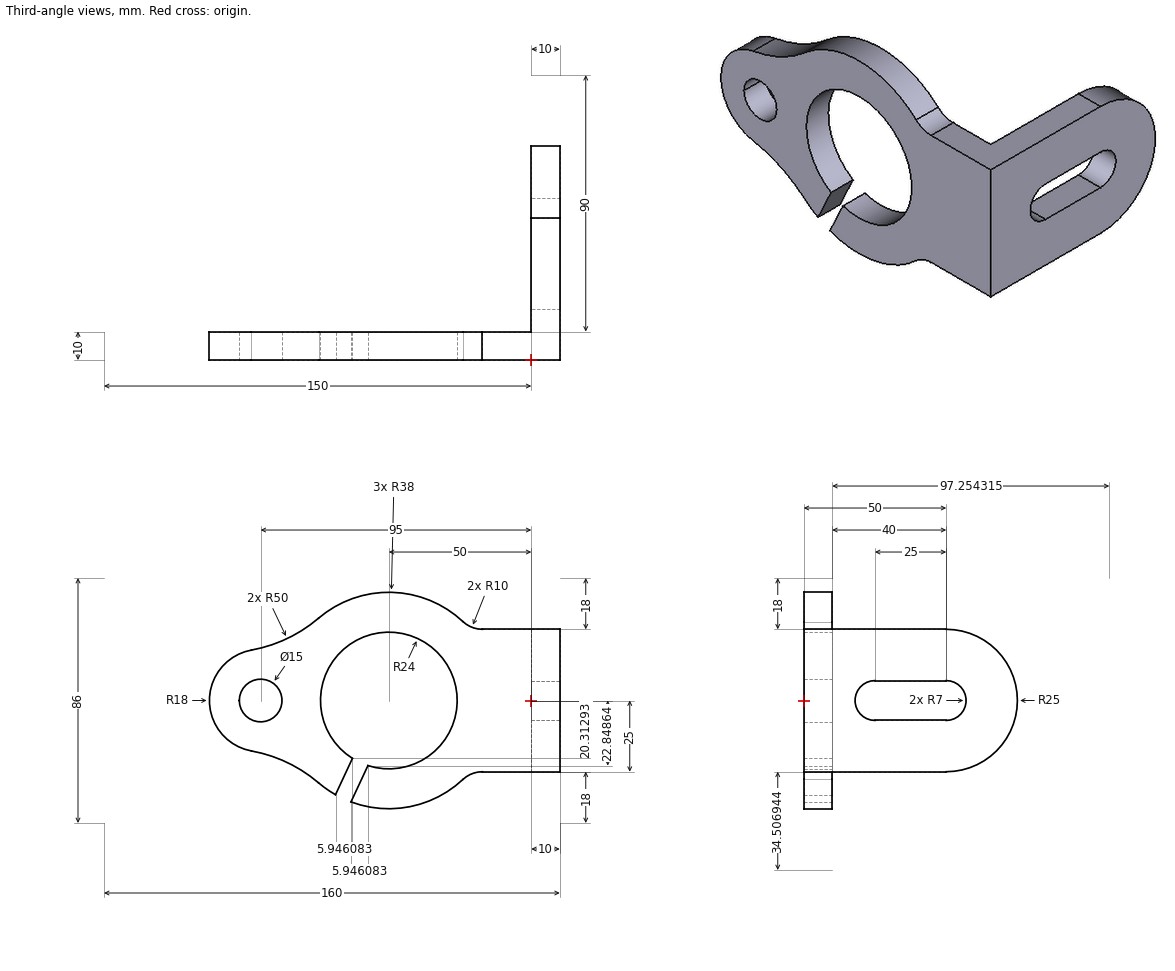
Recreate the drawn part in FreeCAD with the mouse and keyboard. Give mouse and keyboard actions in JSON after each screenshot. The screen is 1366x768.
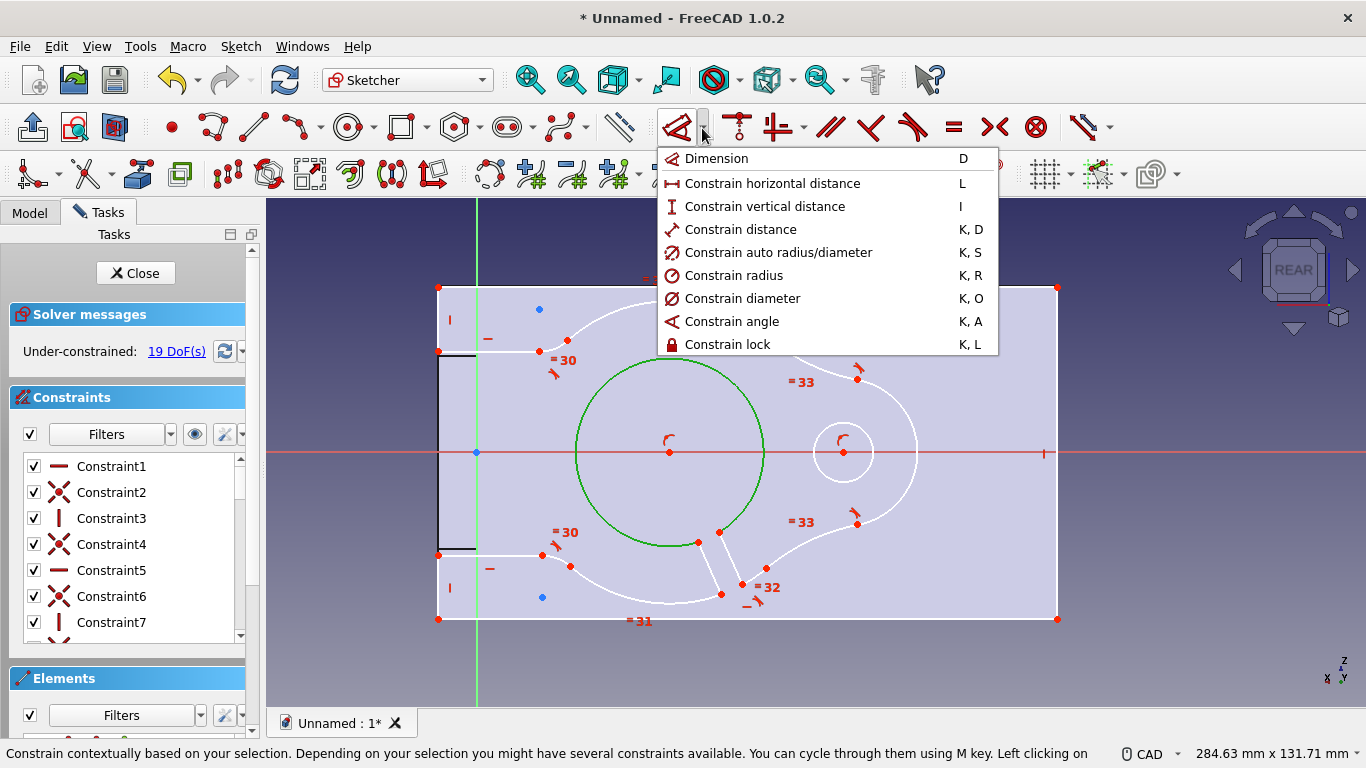
{"action": "left_click", "coordinate": [828, 276]}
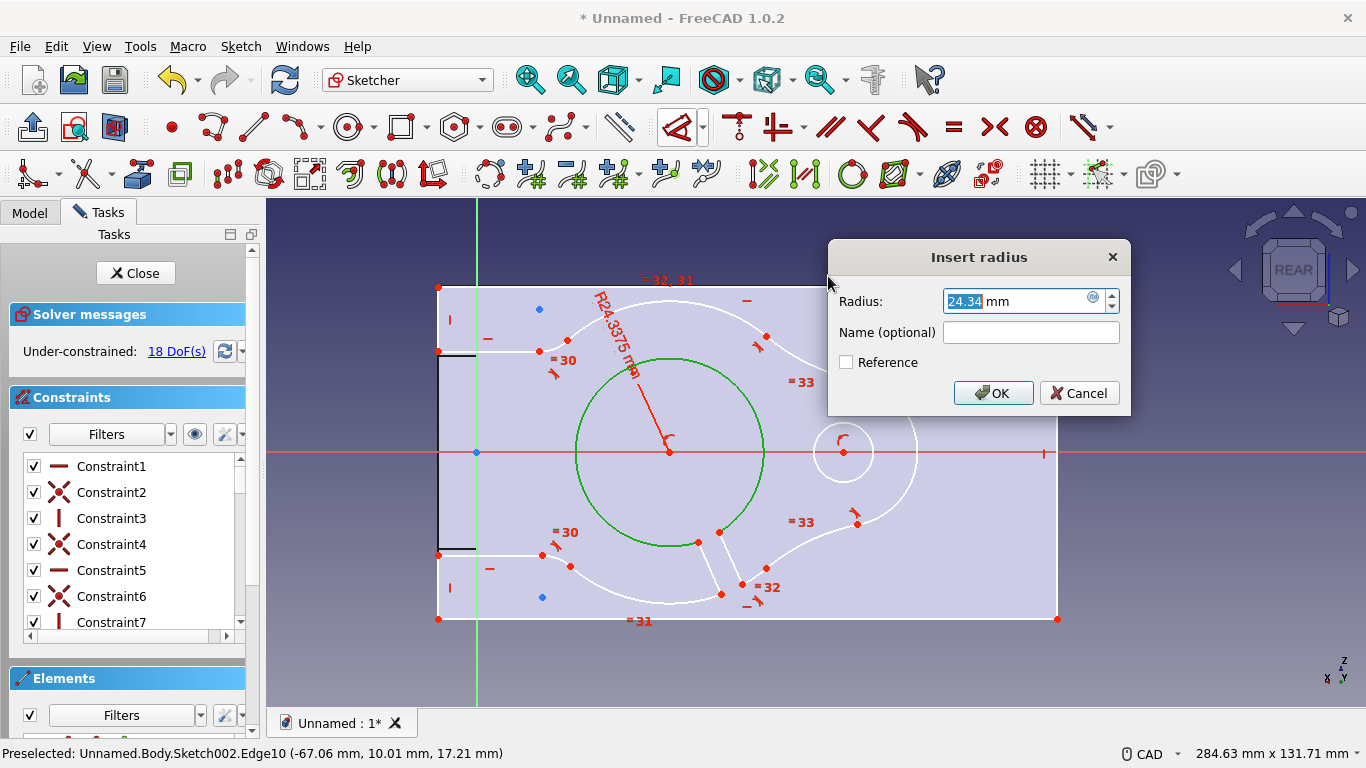
{"action": "type", "text": "24"}
{"action": "key", "text": "Return"}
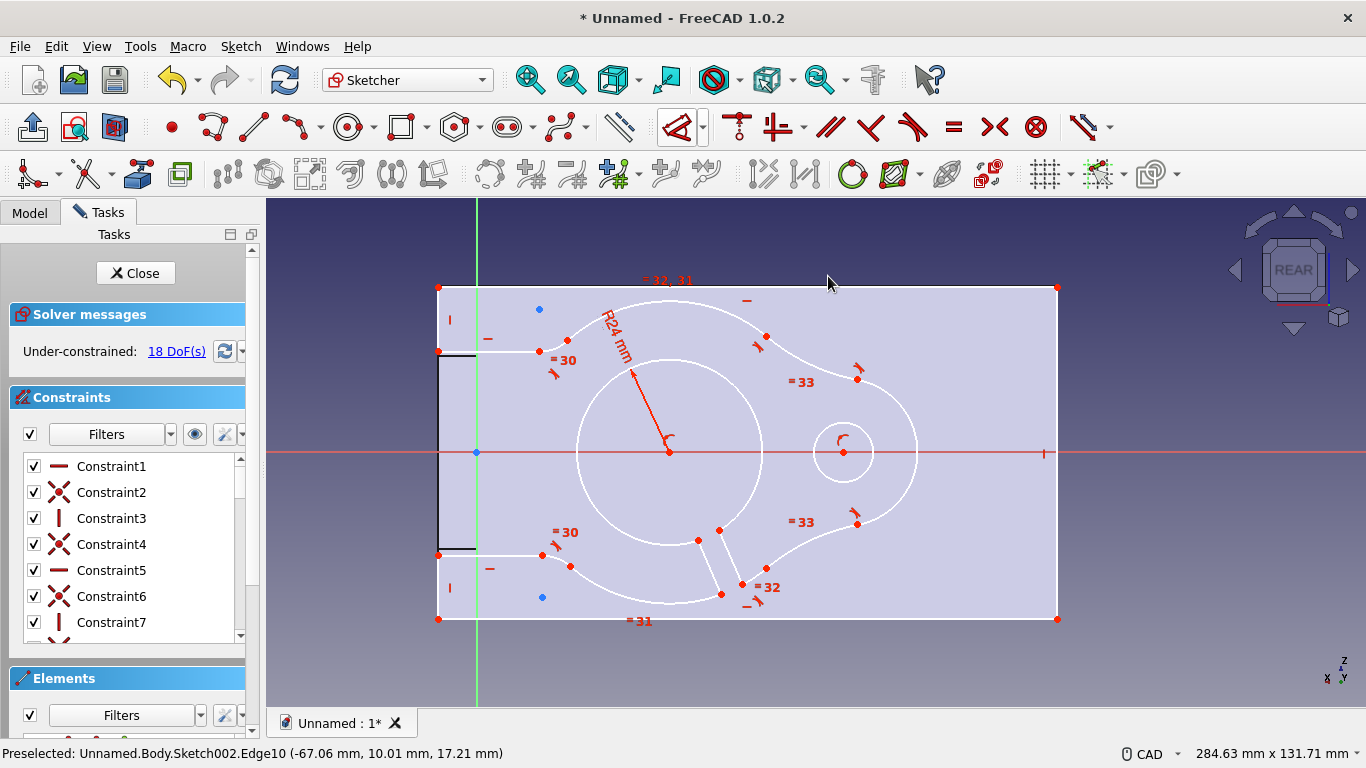
{"action": "left_click", "coordinate": [611, 592]}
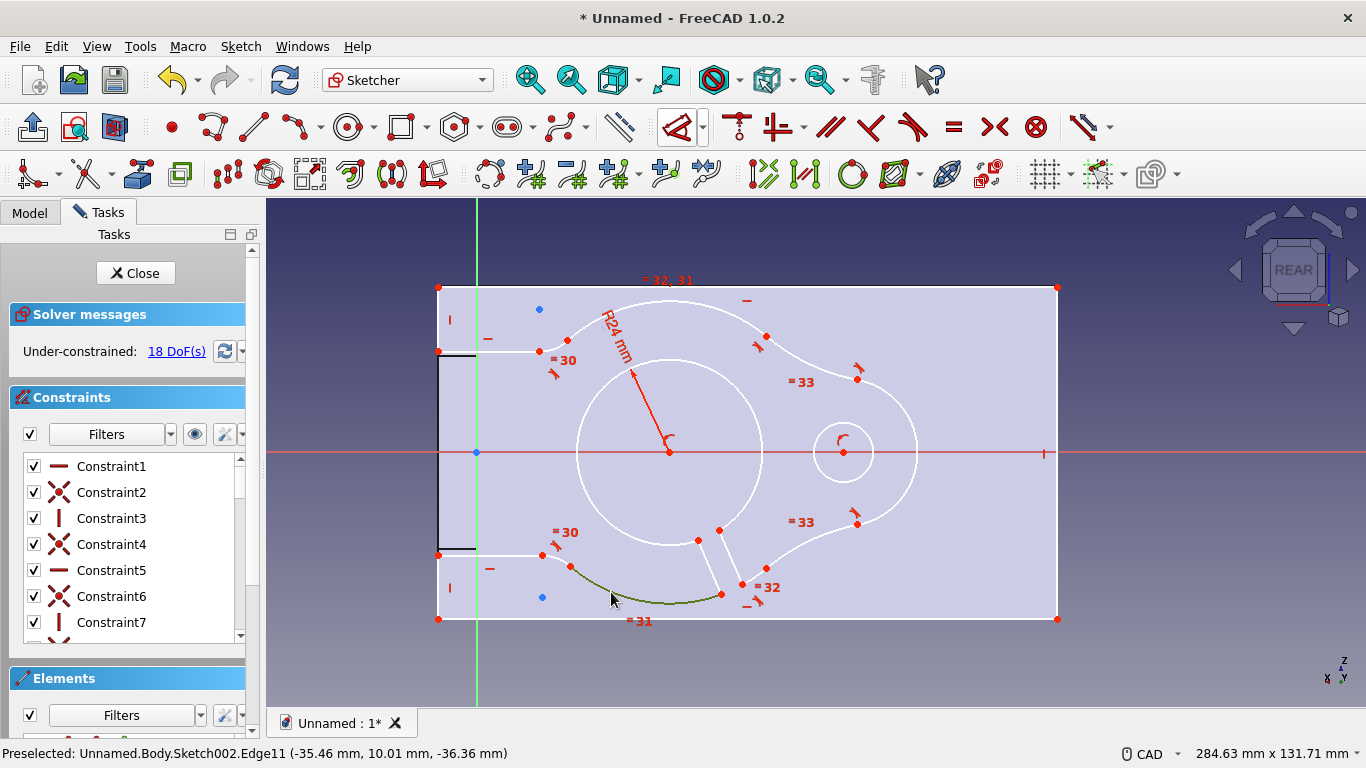
{"action": "key", "text": "k r"}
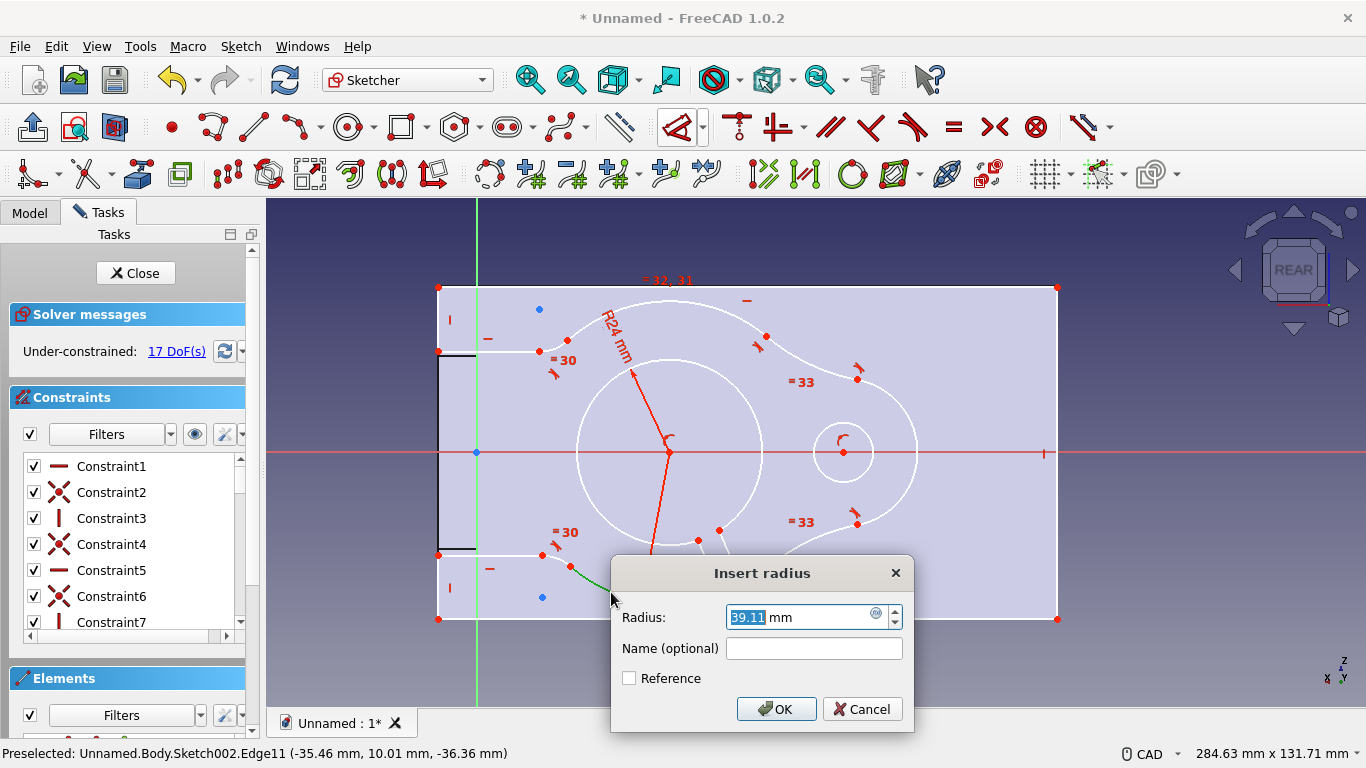
{"action": "type", "text": "38"}
{"action": "key", "text": "Return"}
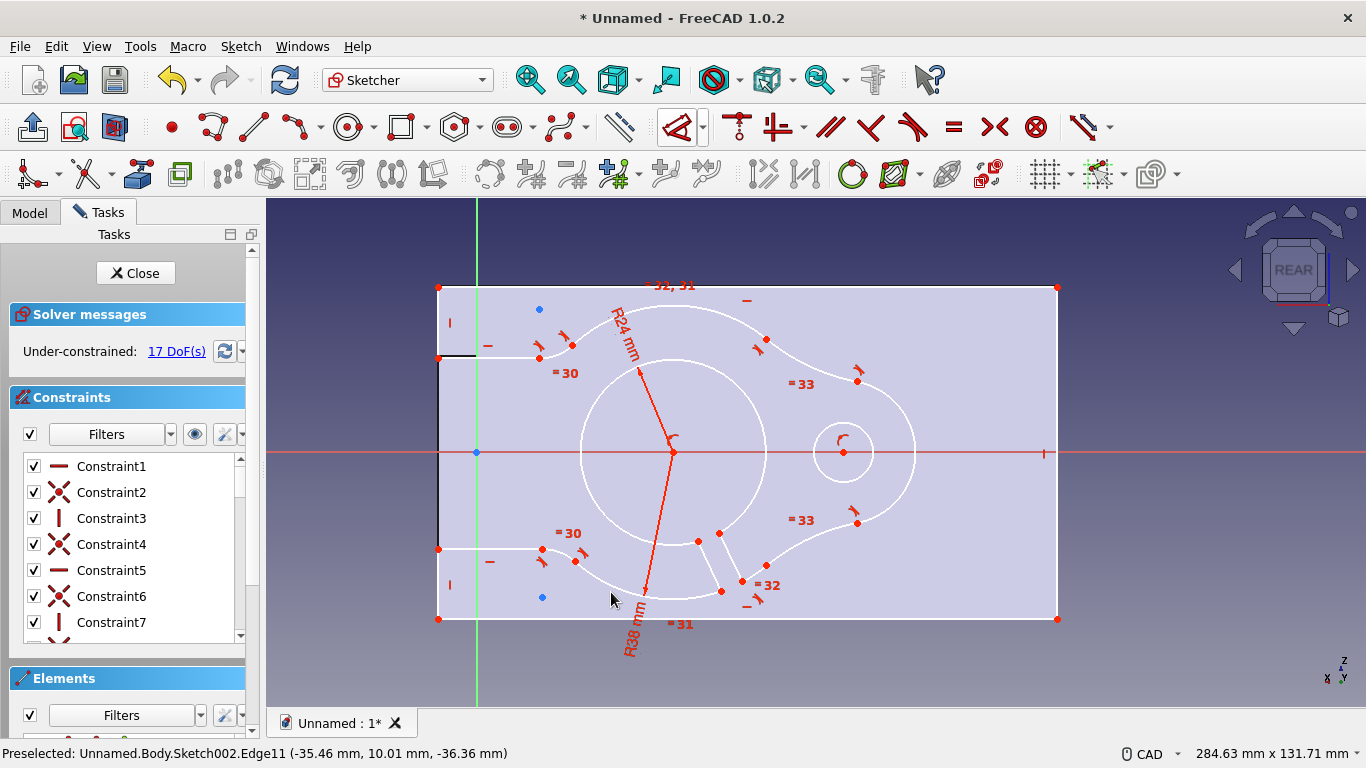
{"action": "scroll", "coordinate": [566, 555], "scroll_direction": "up", "scroll_amount": 2}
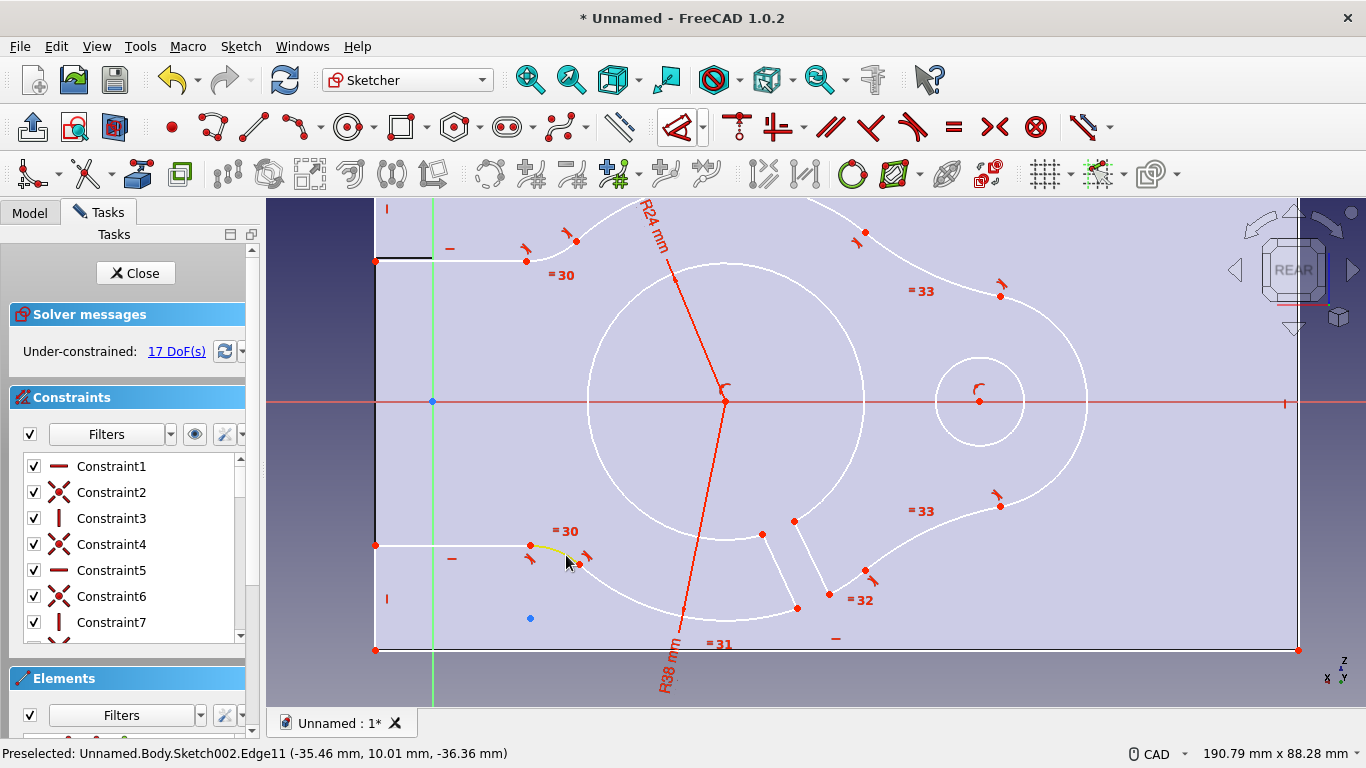
{"action": "left_click", "coordinate": [566, 555]}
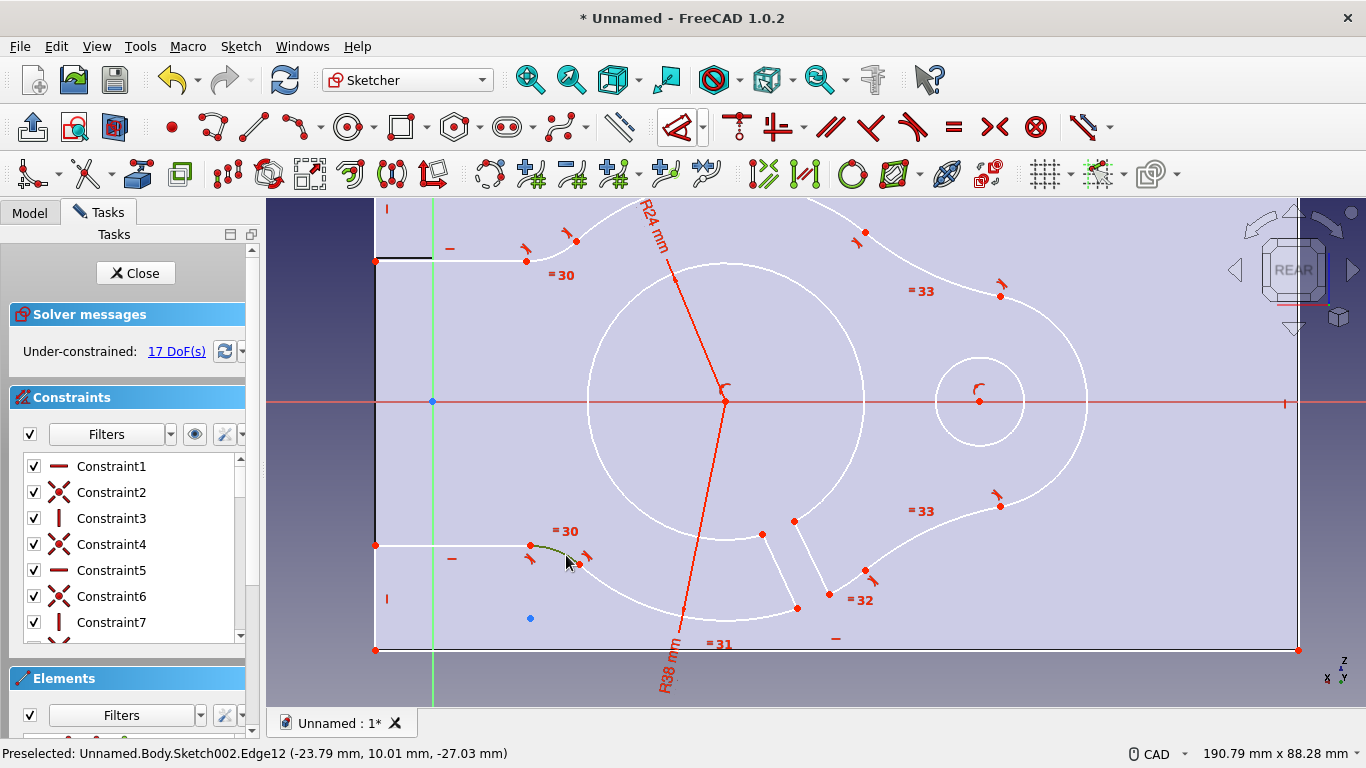
{"action": "key", "text": "k r"}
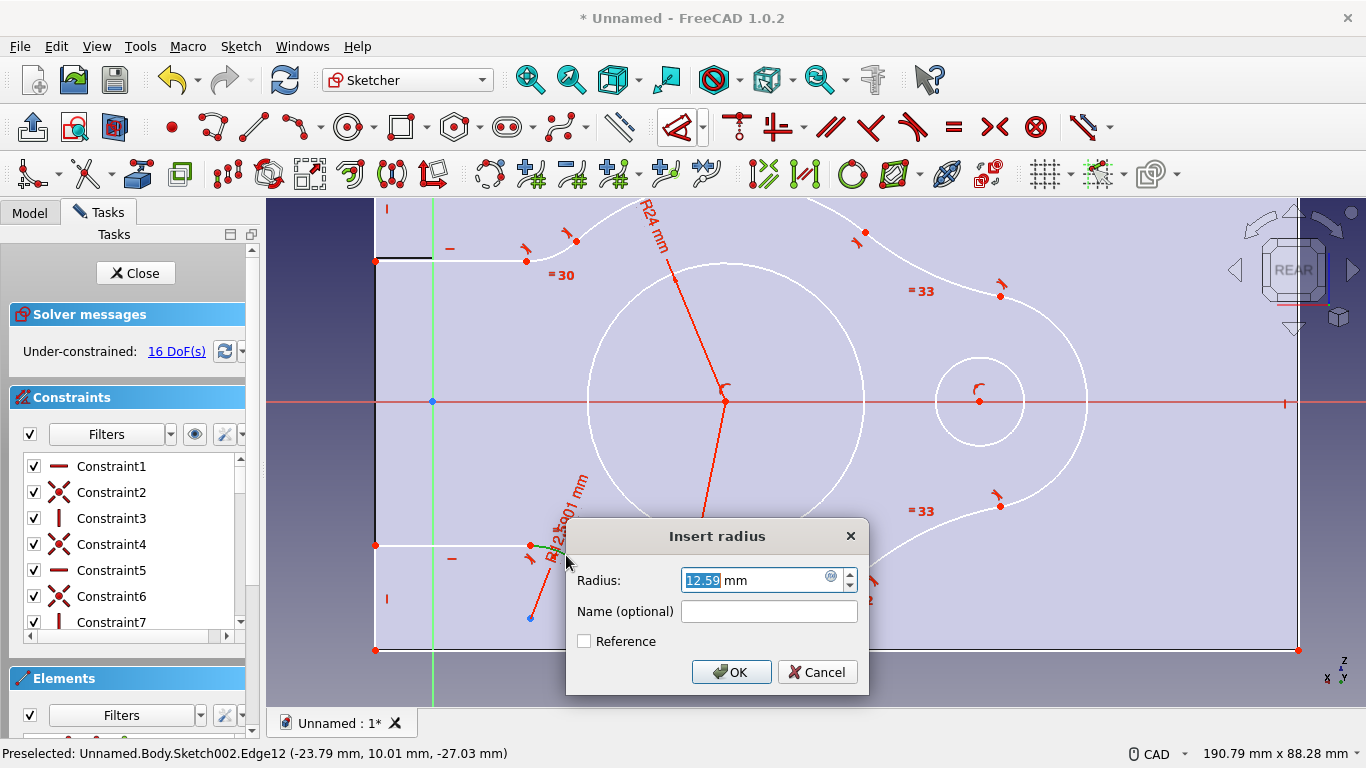
{"action": "type", "text": "10"}
{"action": "key", "text": "Return"}